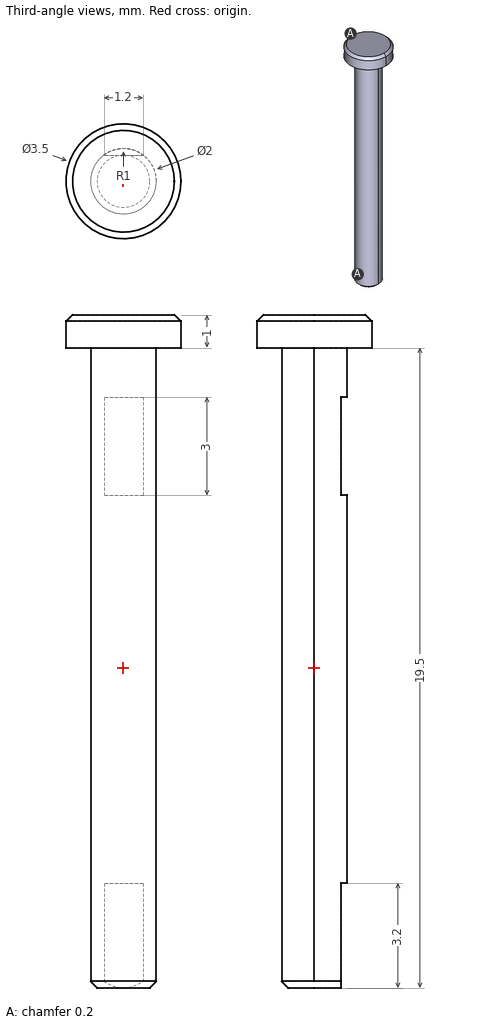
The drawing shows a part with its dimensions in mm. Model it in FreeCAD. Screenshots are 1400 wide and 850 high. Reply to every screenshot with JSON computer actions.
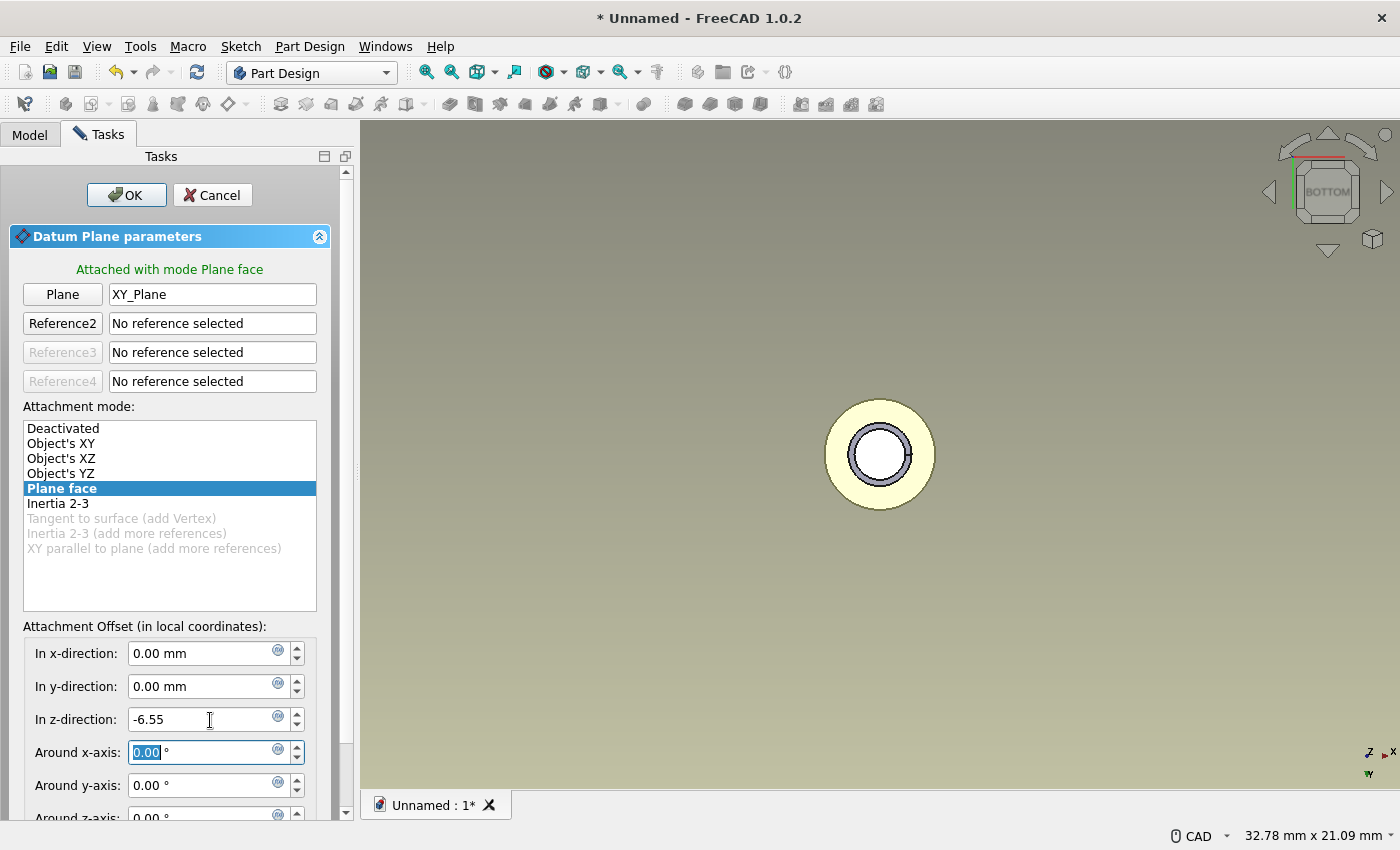
{"action": "left_click", "coordinate": [127, 195]}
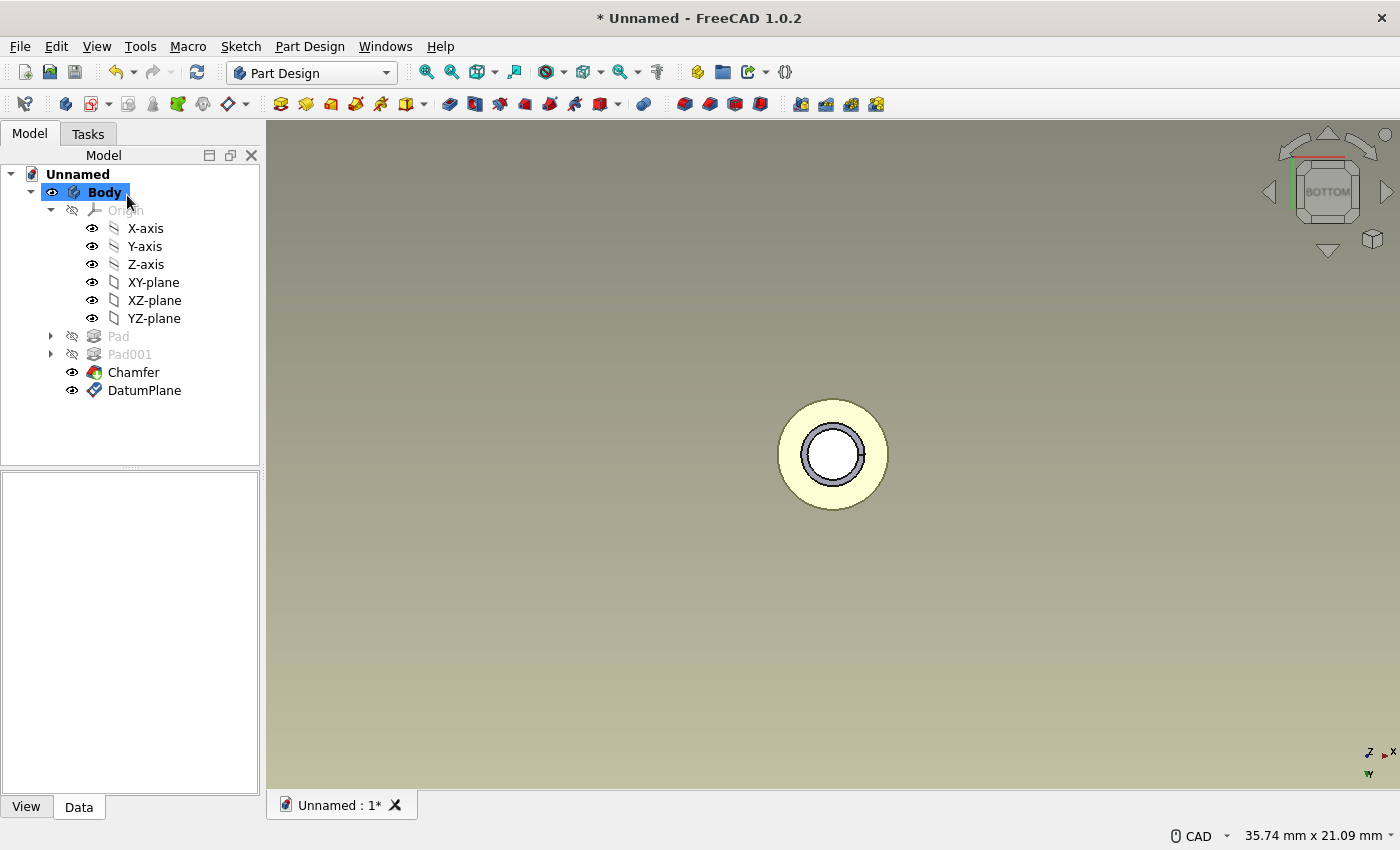
{"action": "left_click", "coordinate": [117, 390]}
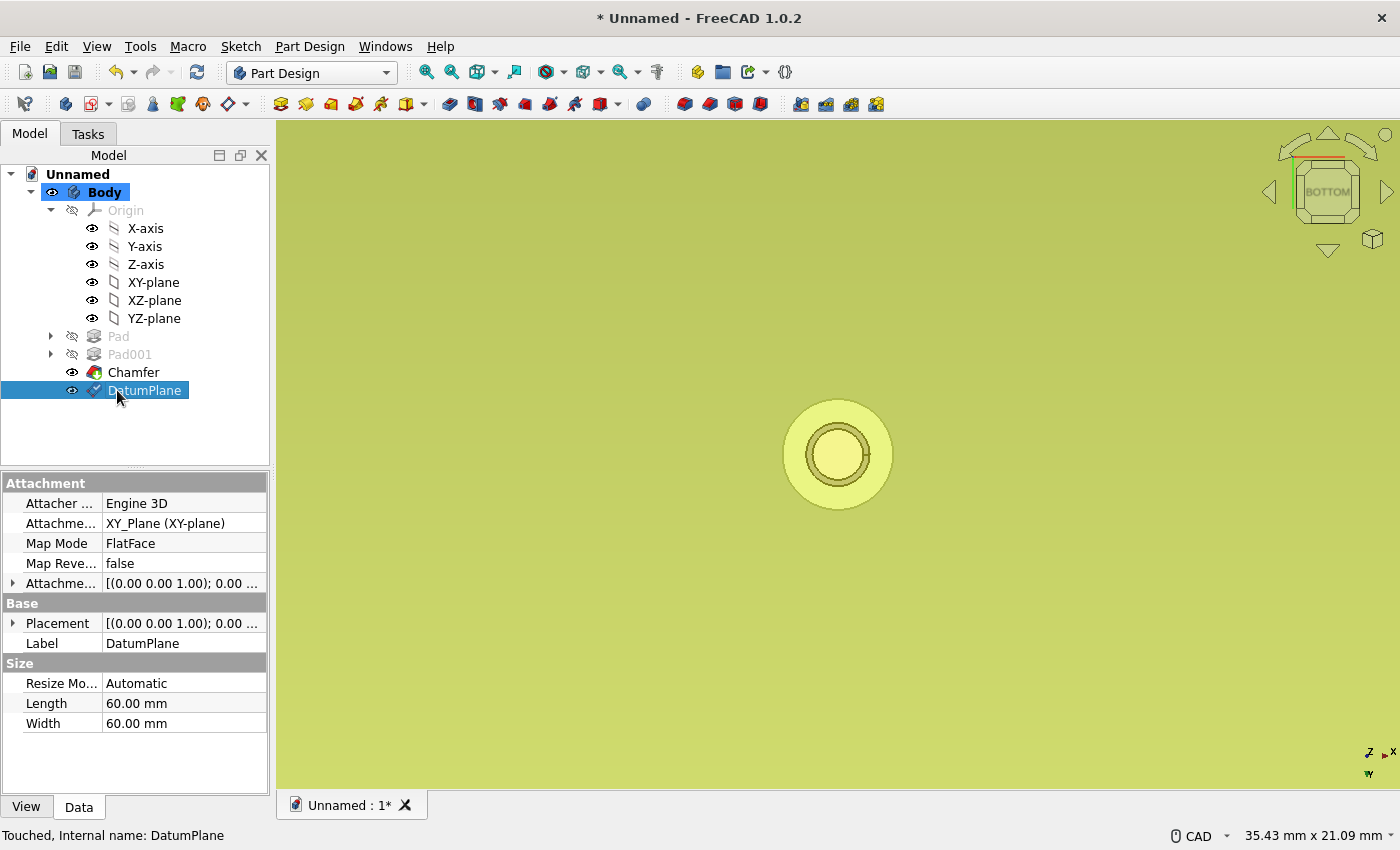
{"action": "left_click", "coordinate": [90, 104]}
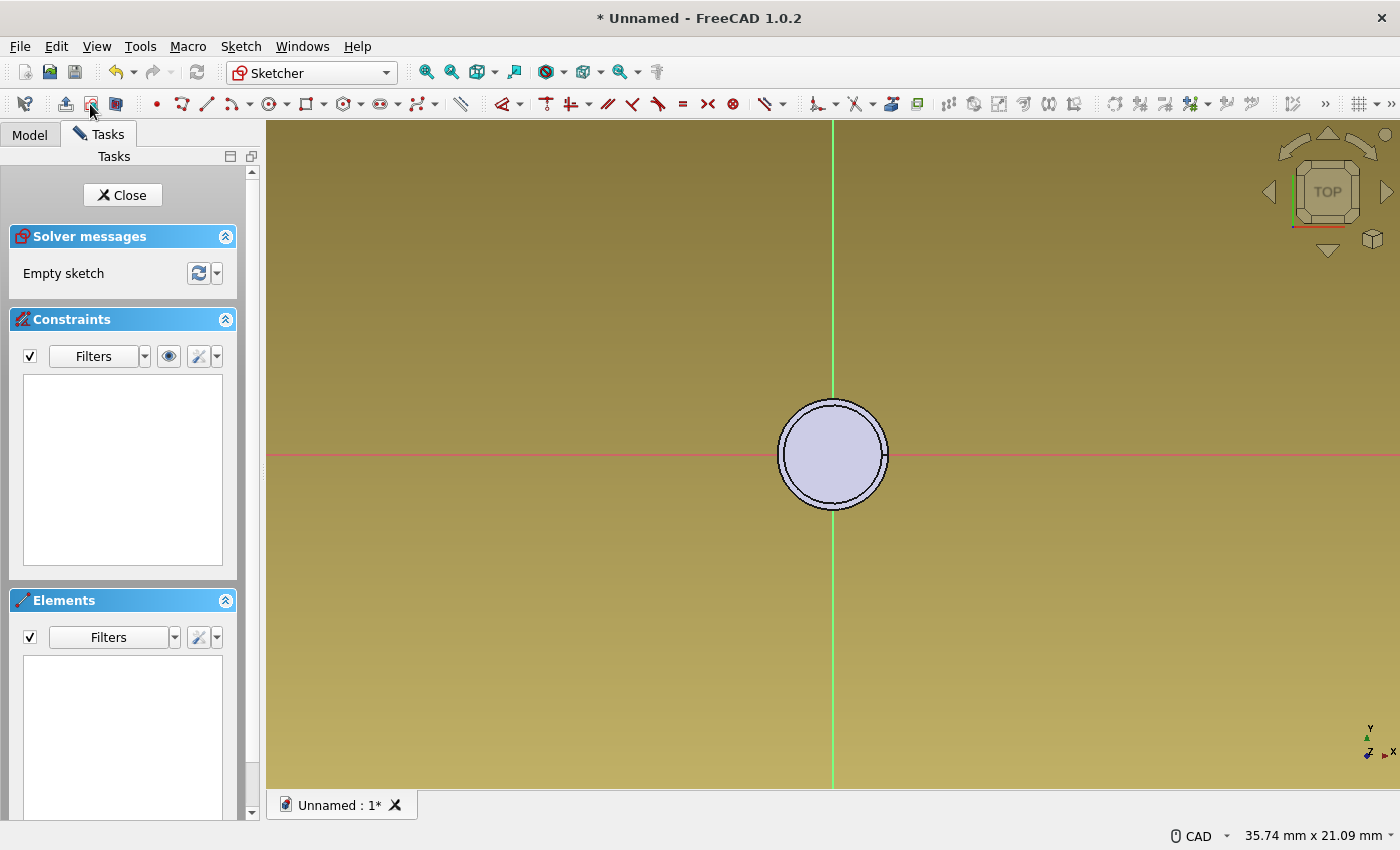
{"action": "left_click", "coordinate": [116, 104]}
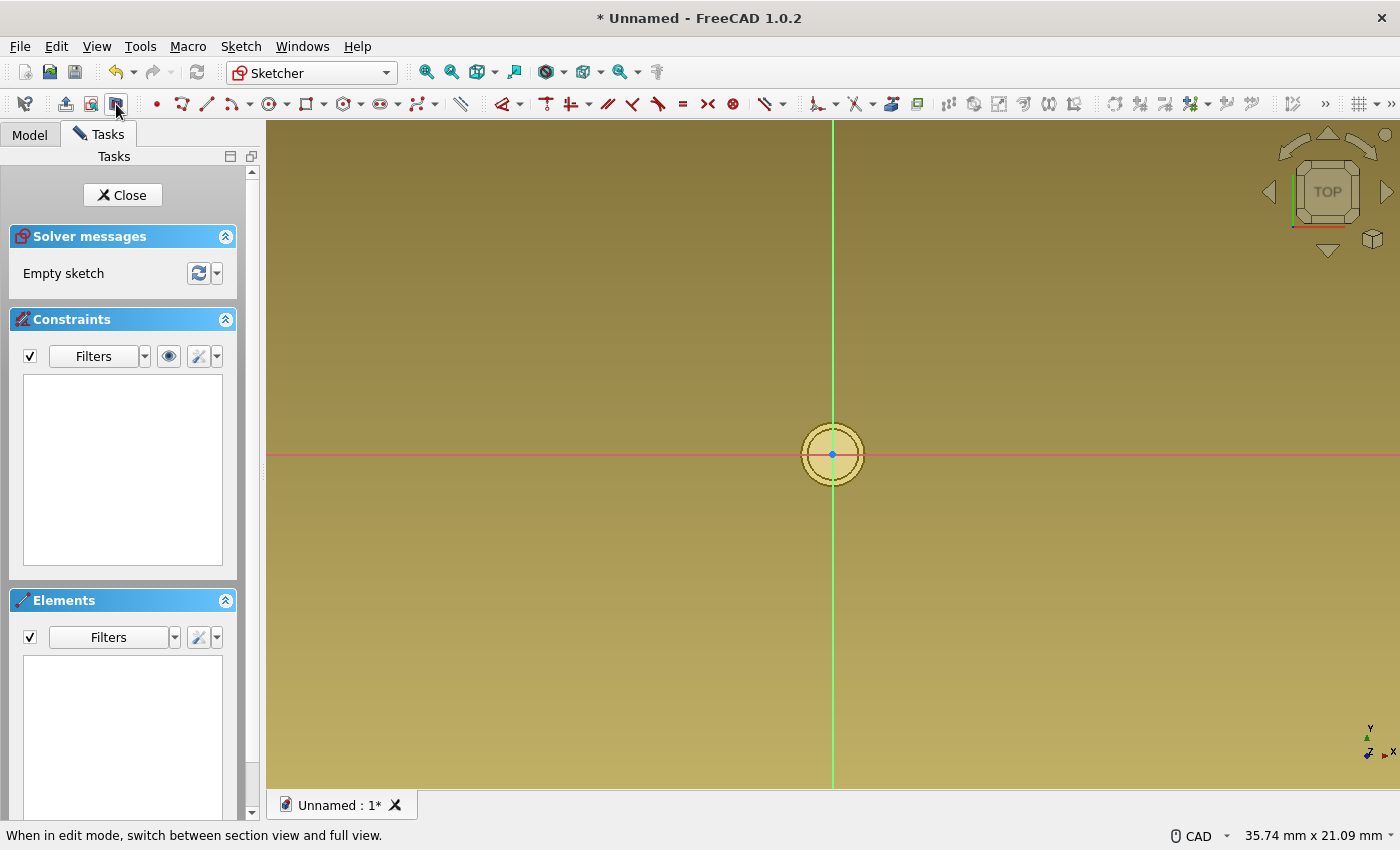
{"action": "scroll", "coordinate": [838, 437], "scroll_direction": "up", "scroll_amount": 13}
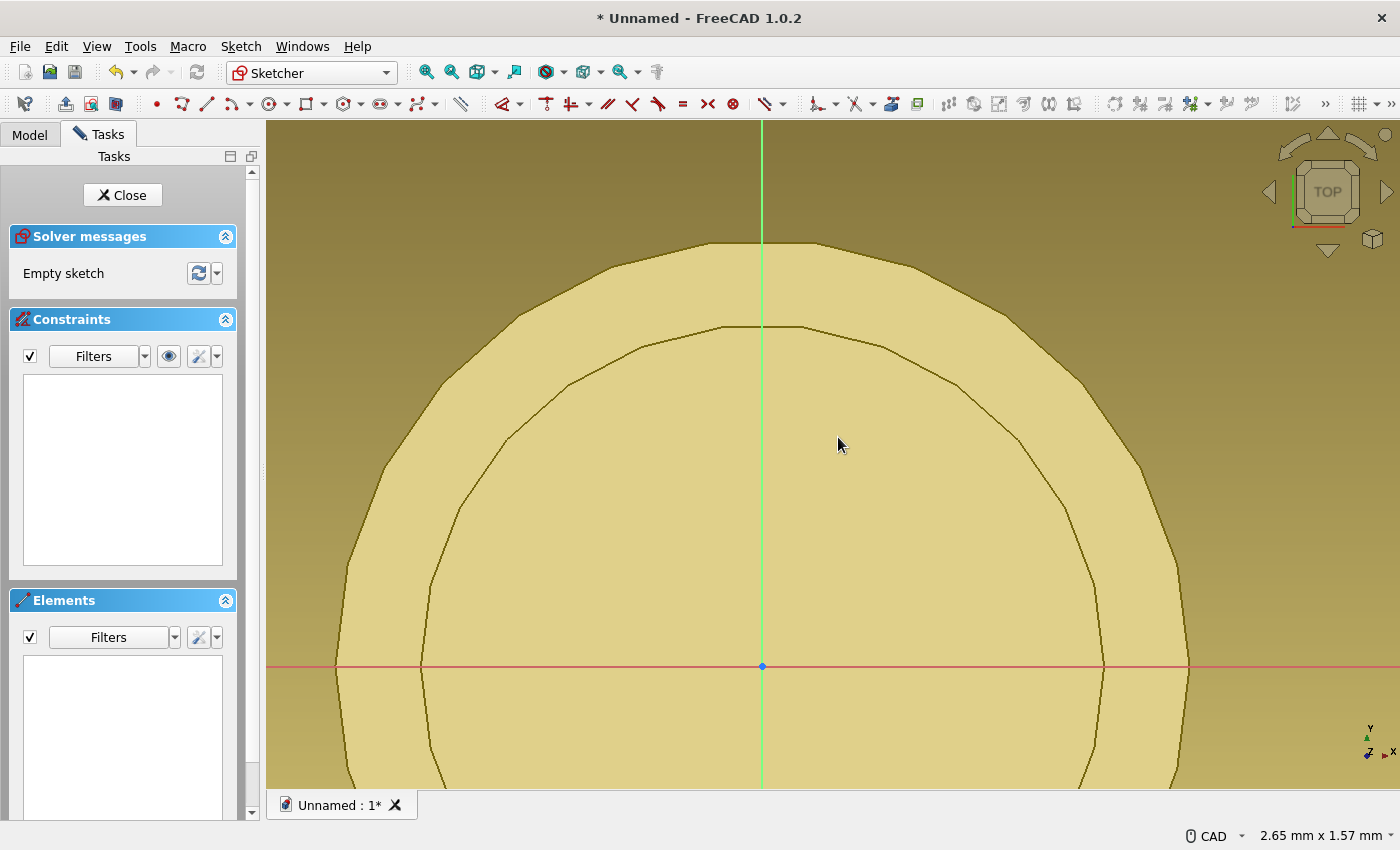
{"action": "left_click", "coordinate": [207, 104]}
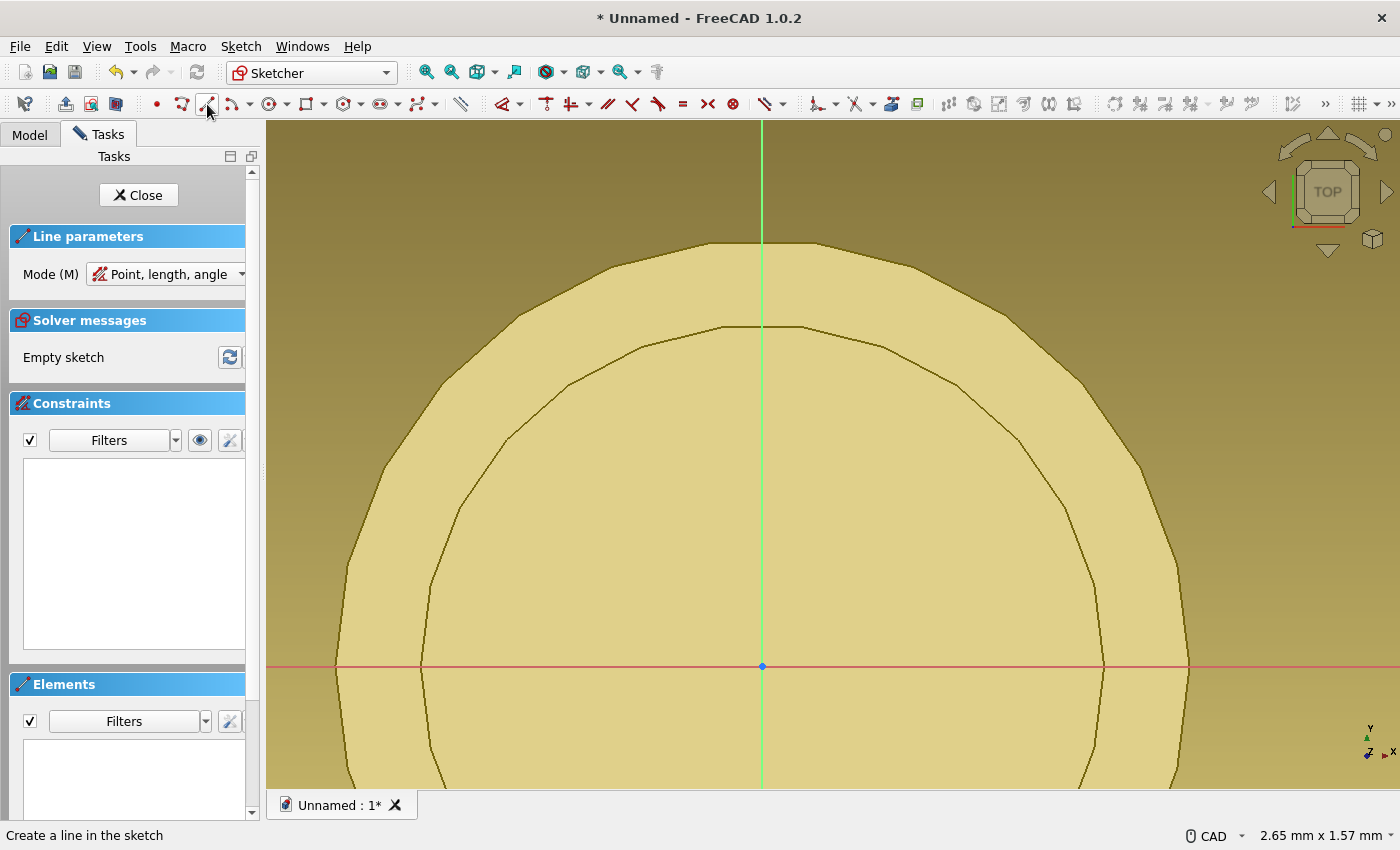
{"action": "left_click", "coordinate": [1019, 325]}
{"action": "left_click", "coordinate": [506, 325]}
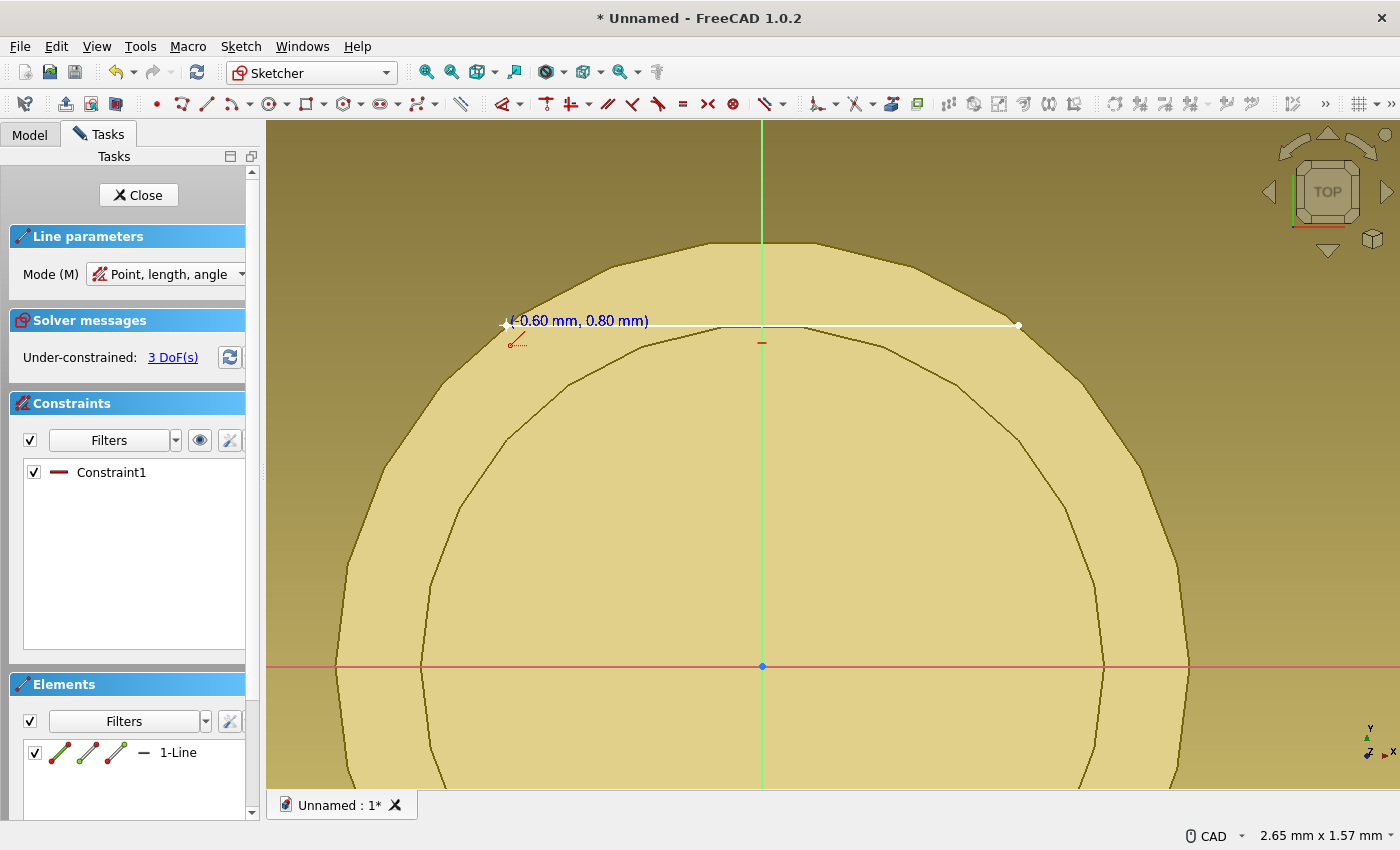
{"action": "key", "text": "g 3 a"}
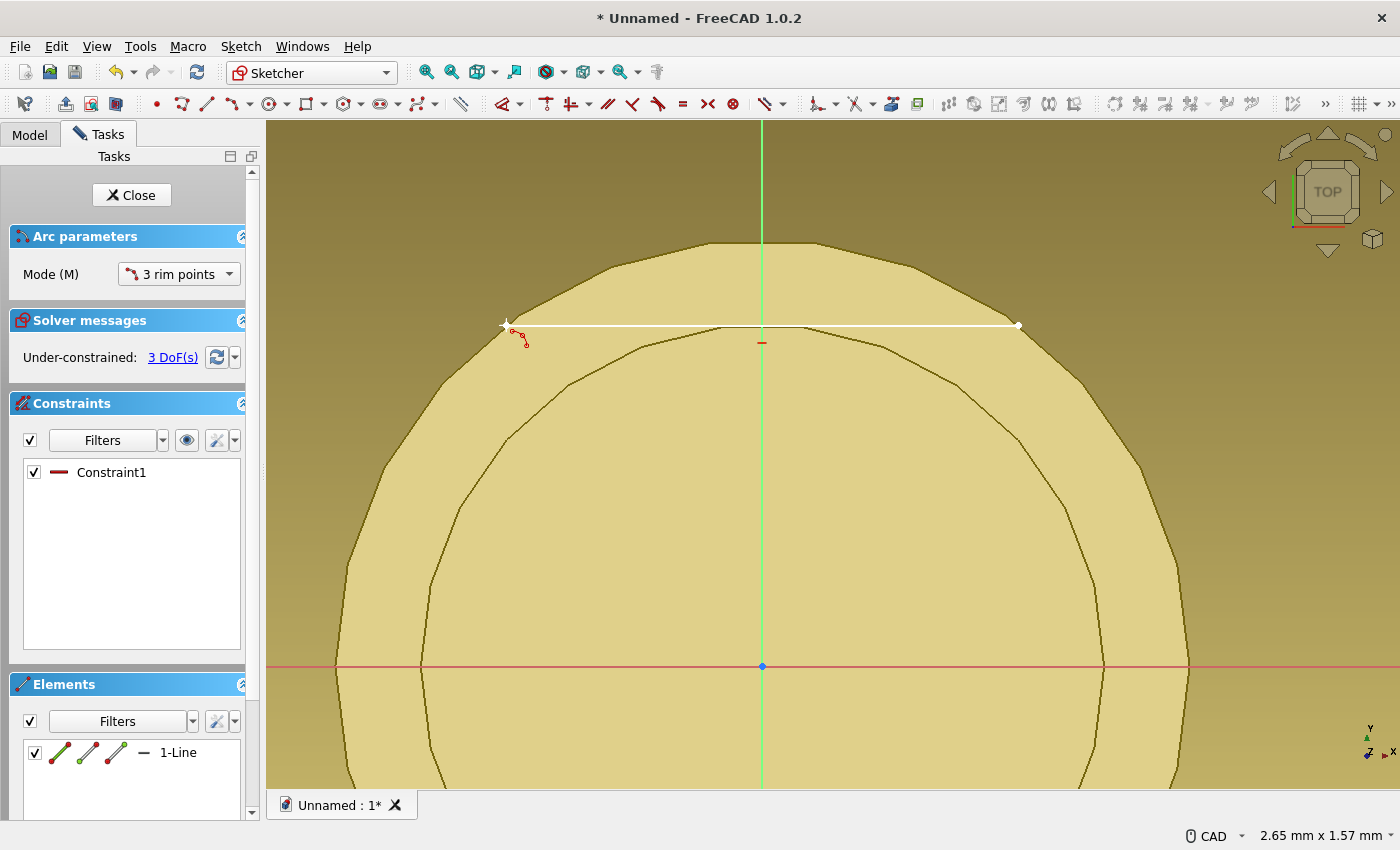
{"action": "left_click", "coordinate": [506, 326]}
{"action": "left_click", "coordinate": [1019, 326]}
{"action": "left_click", "coordinate": [817, 243]}
{"action": "key", "text": "Escape"}